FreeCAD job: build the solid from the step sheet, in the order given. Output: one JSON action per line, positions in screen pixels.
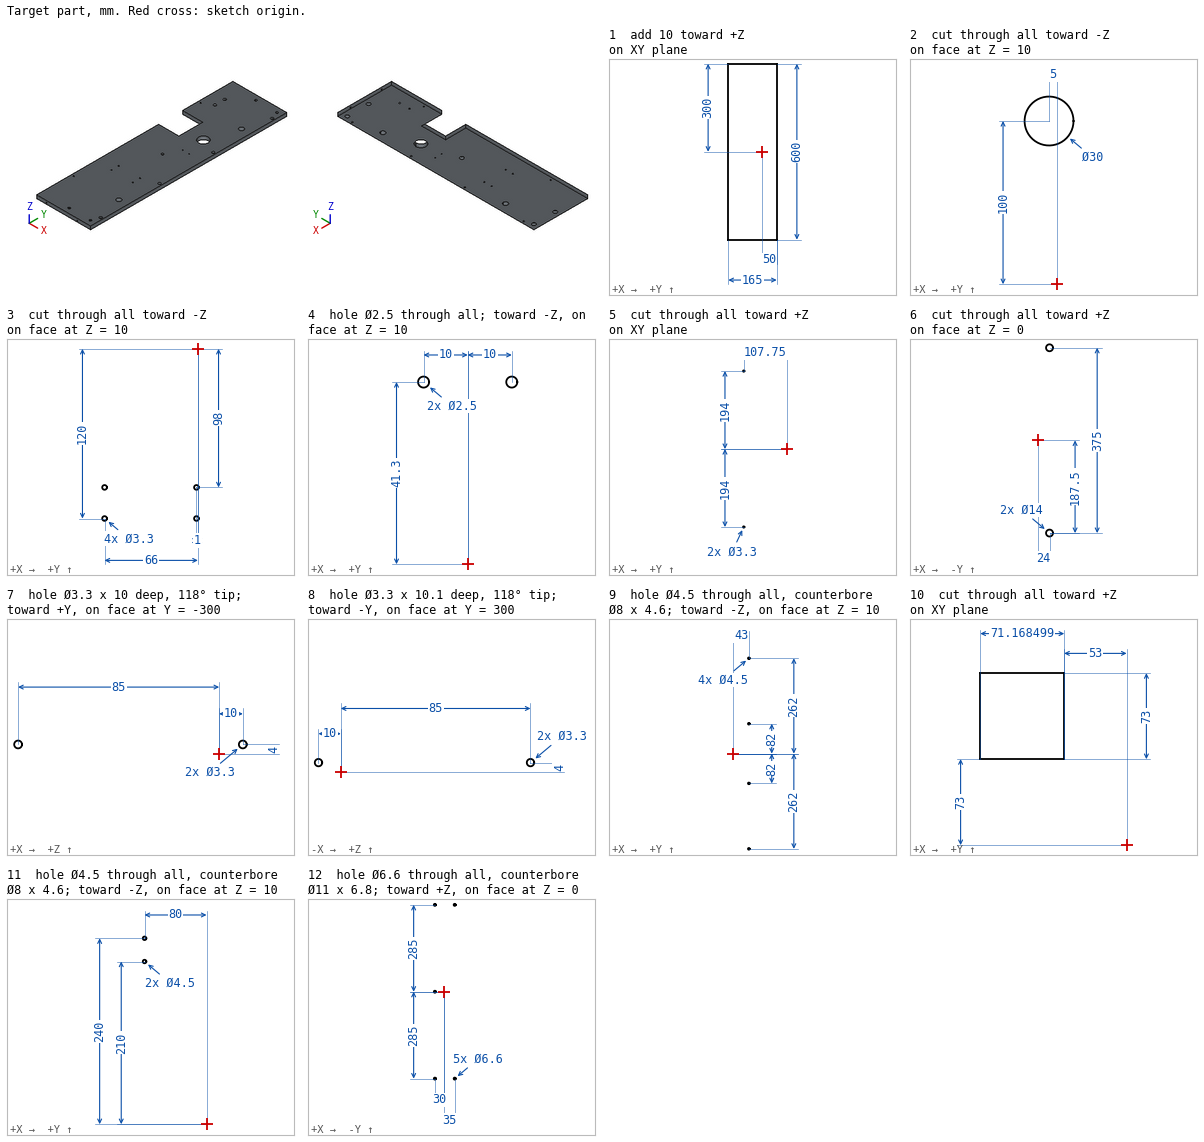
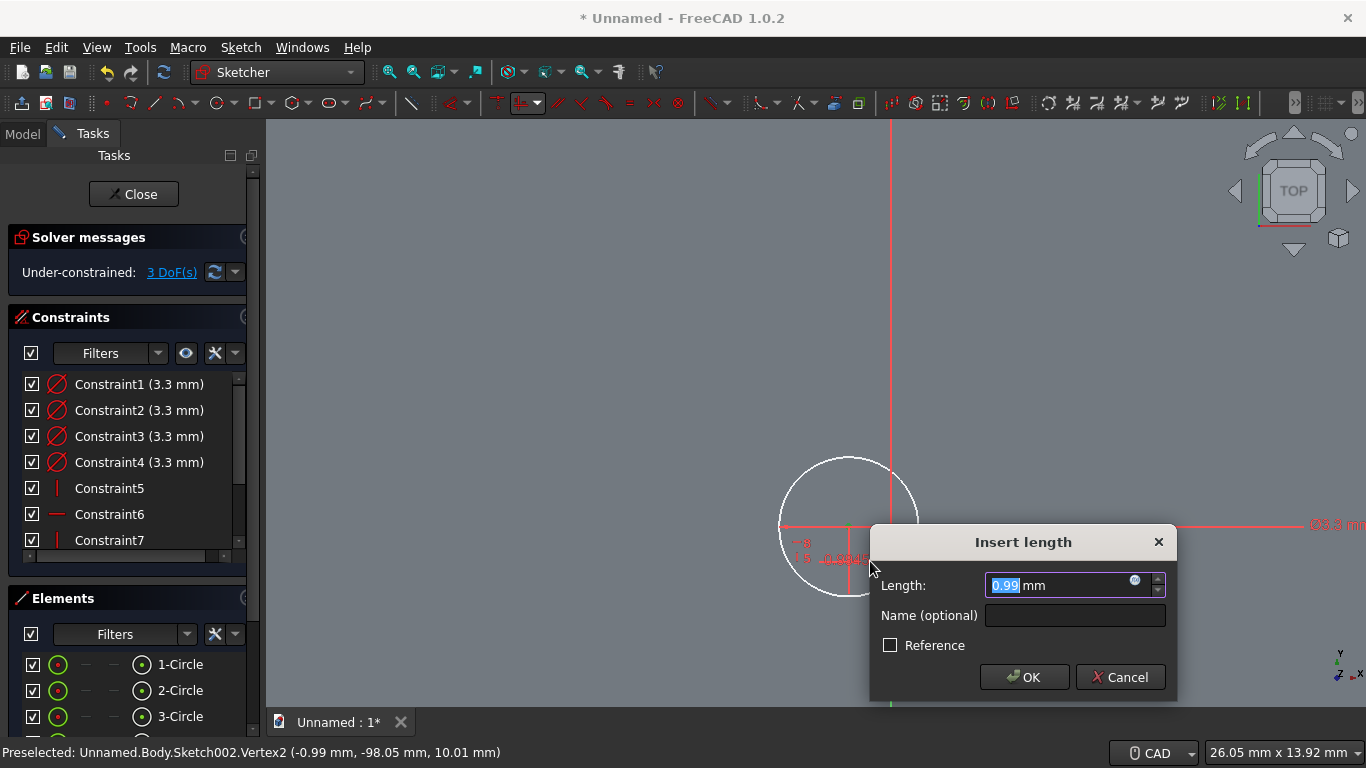
{"action": "type", "text": "1"}
{"action": "key", "text": "Return"}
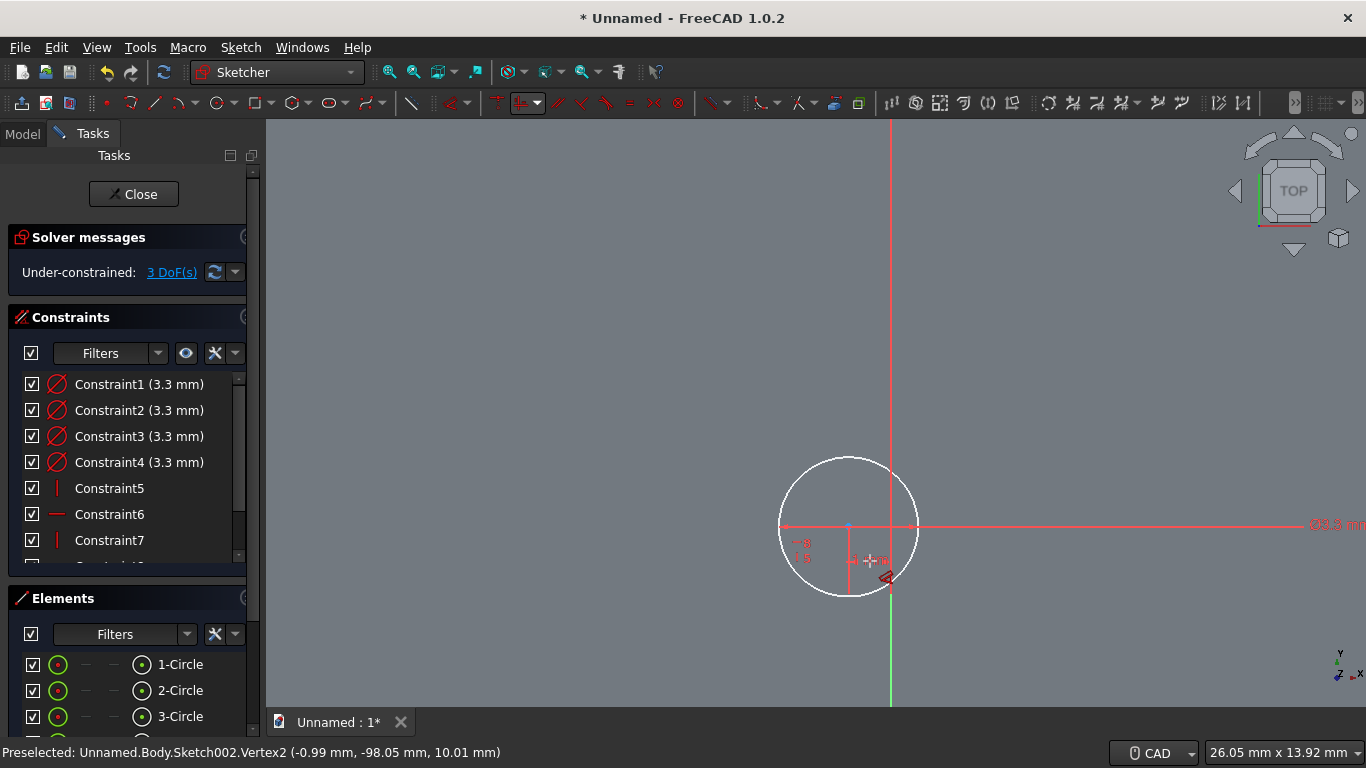
{"action": "scroll", "coordinate": [850, 530], "scroll_direction": "down", "scroll_amount": 13}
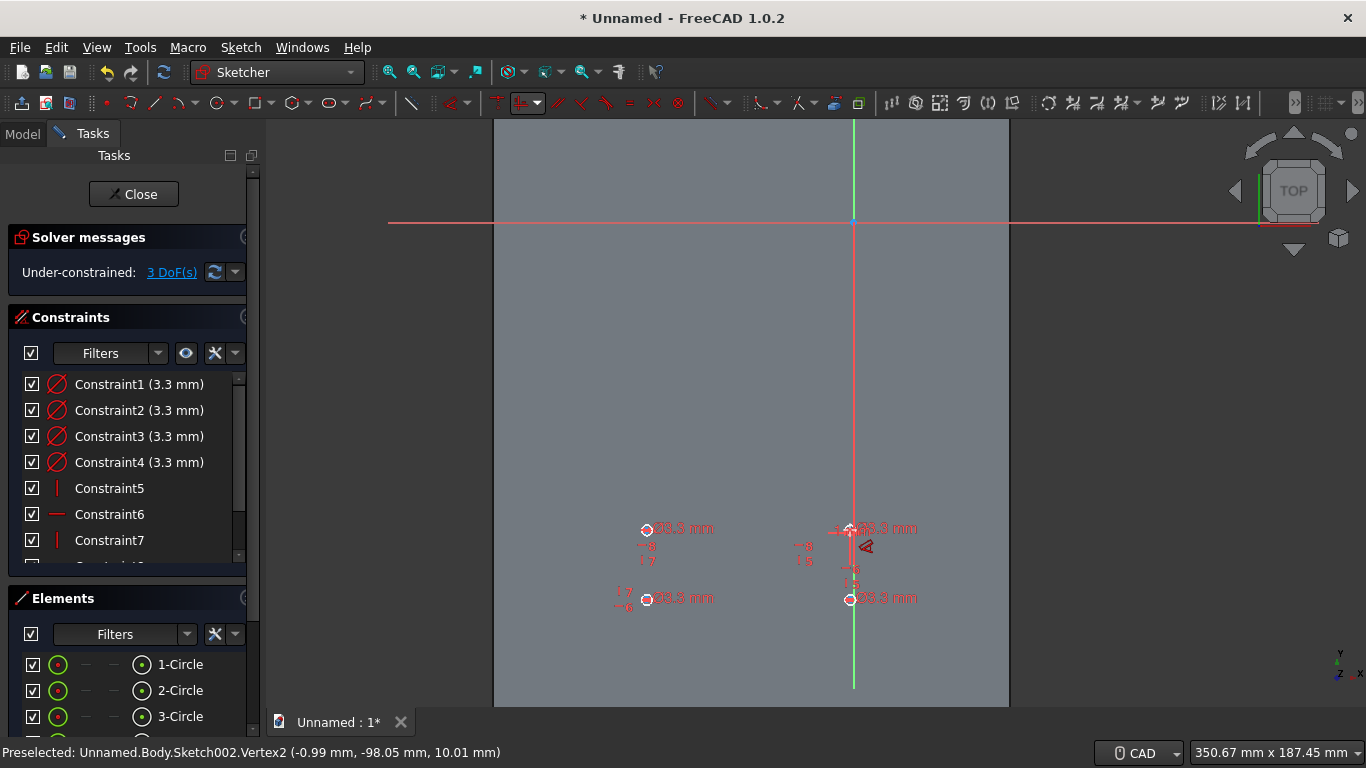
{"action": "left_click", "coordinate": [647, 600]}
{"action": "left_click", "coordinate": [750, 189]}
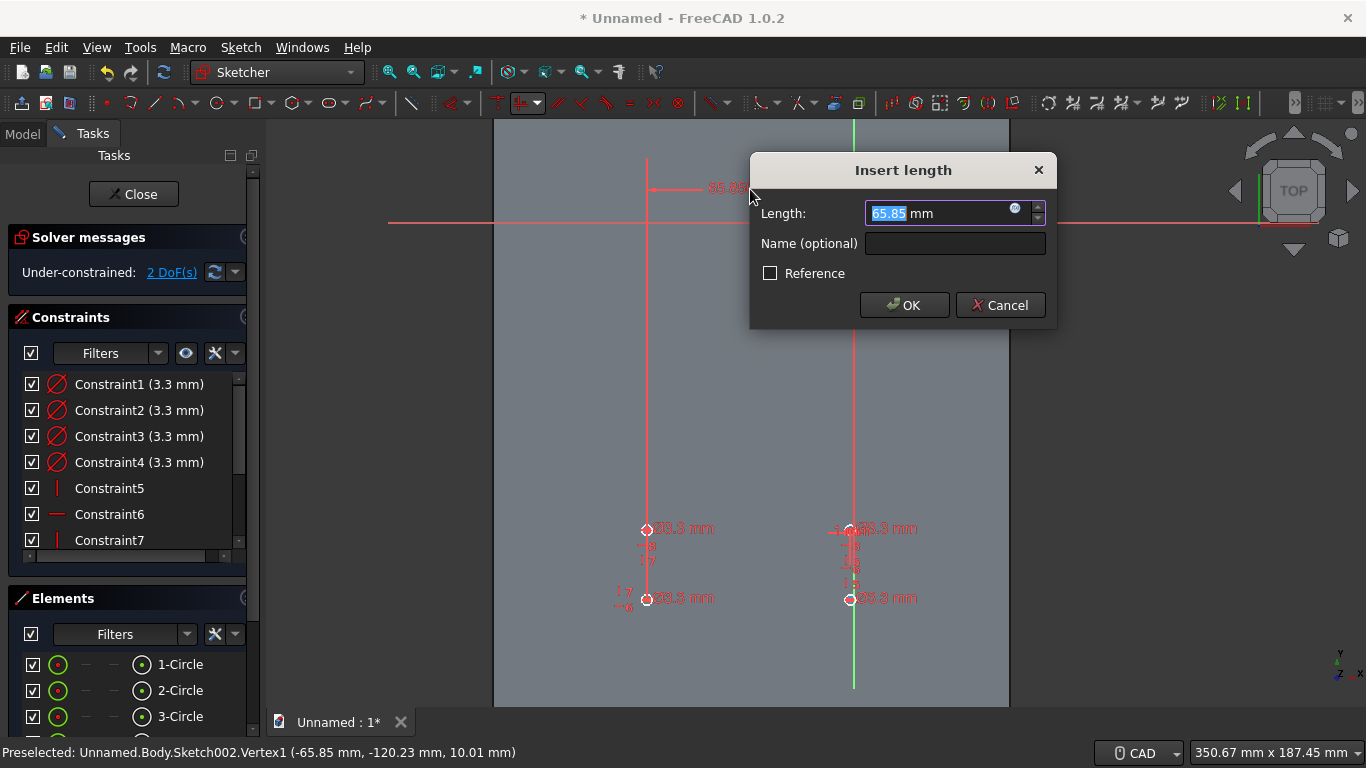
{"action": "type", "text": "66"}
{"action": "key", "text": "Return"}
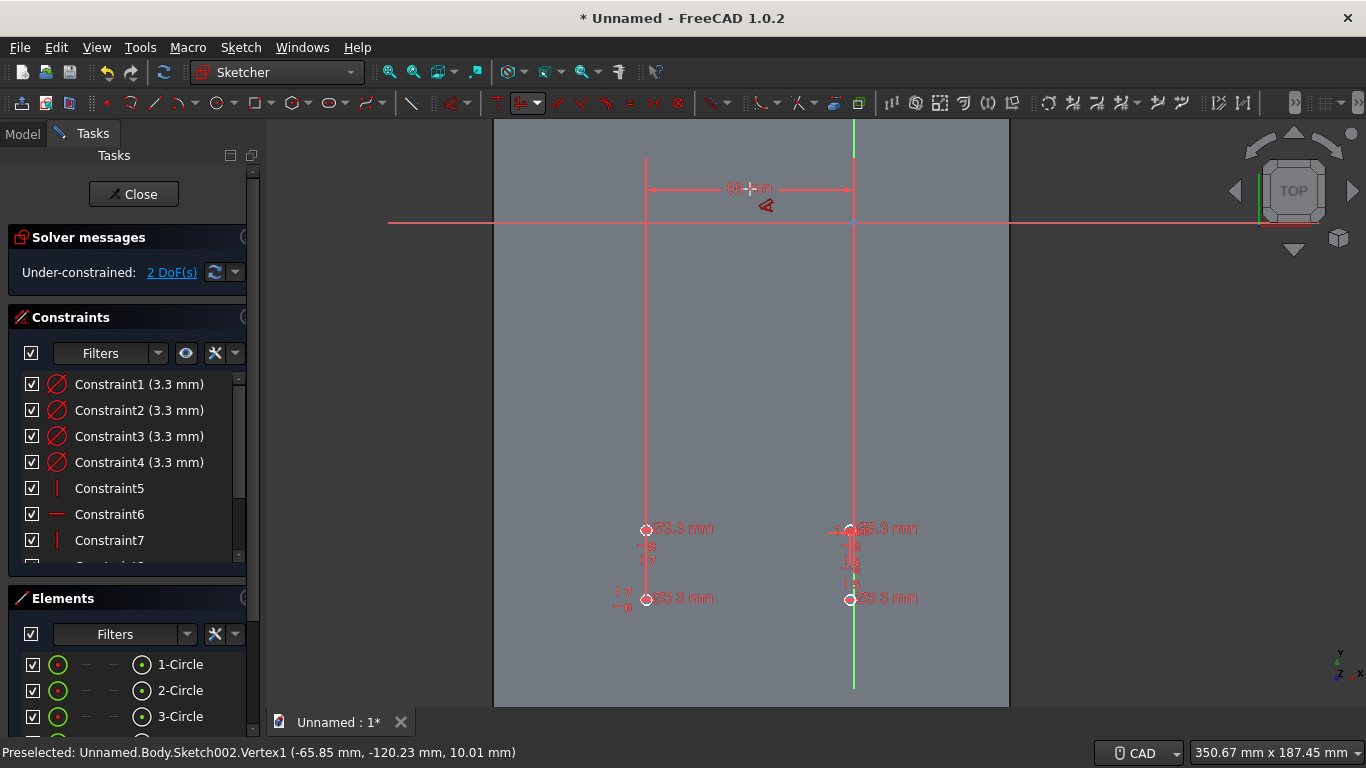
{"action": "left_click", "coordinate": [850, 530]}
{"action": "left_click", "coordinate": [888, 377]}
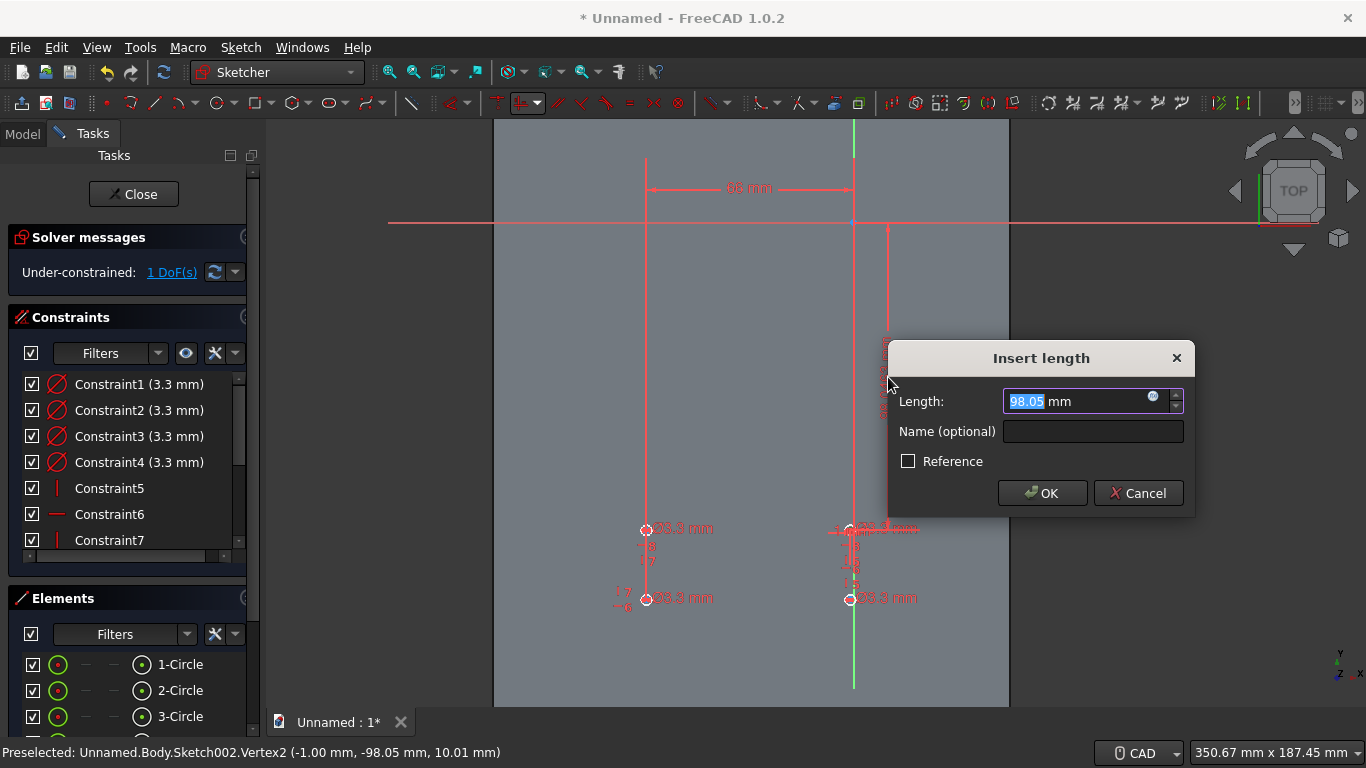
{"action": "type", "text": "98"}
{"action": "key", "text": "Return"}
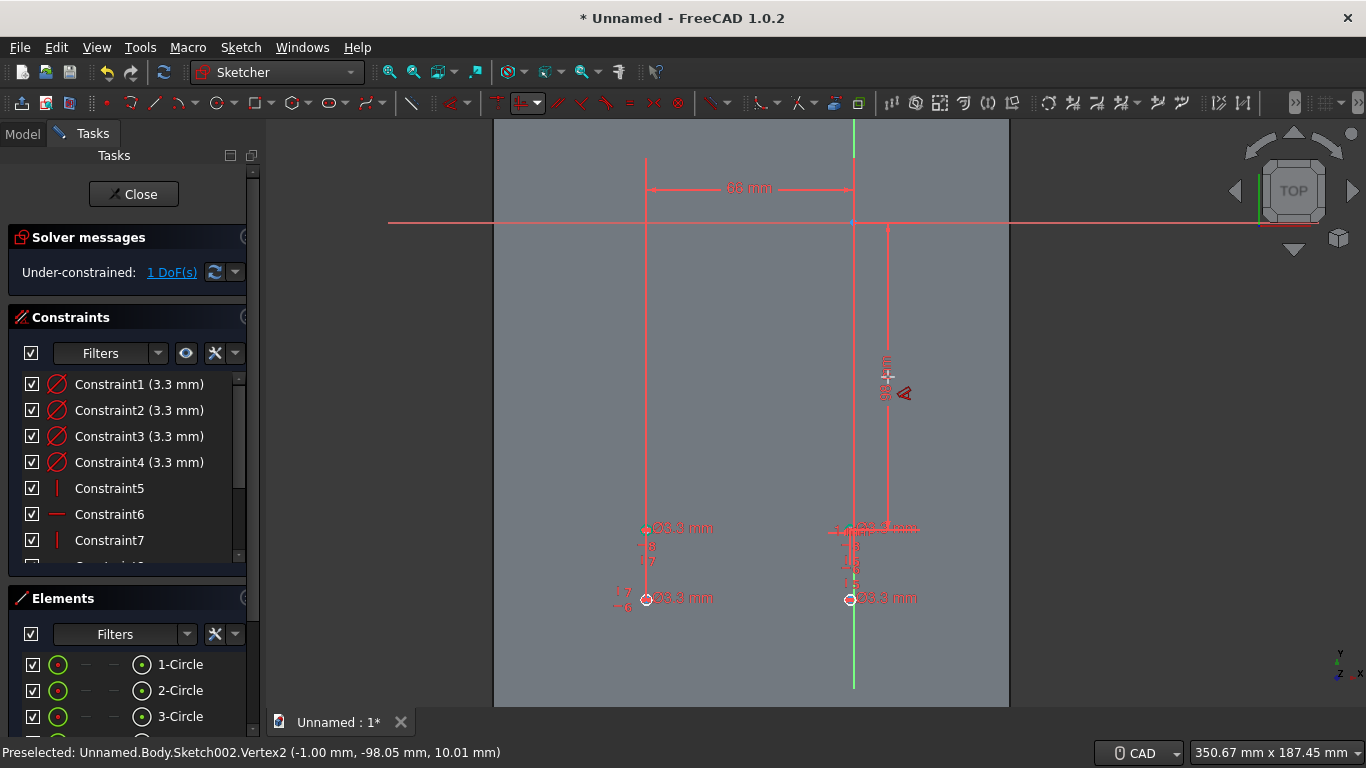
{"action": "left_click", "coordinate": [646, 600]}
{"action": "left_click", "coordinate": [888, 411]}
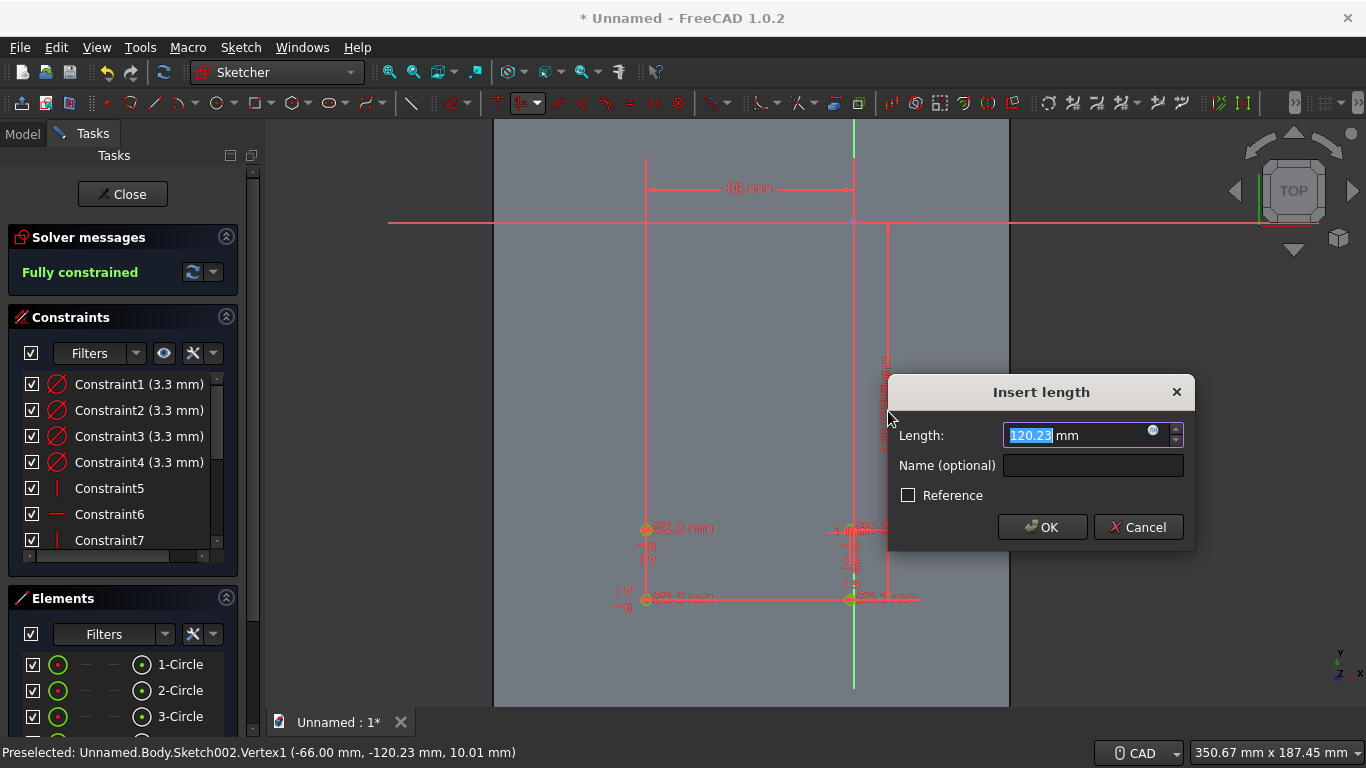
{"action": "type", "text": "120"}
{"action": "key", "text": "Return"}
{"action": "key", "text": "Escape"}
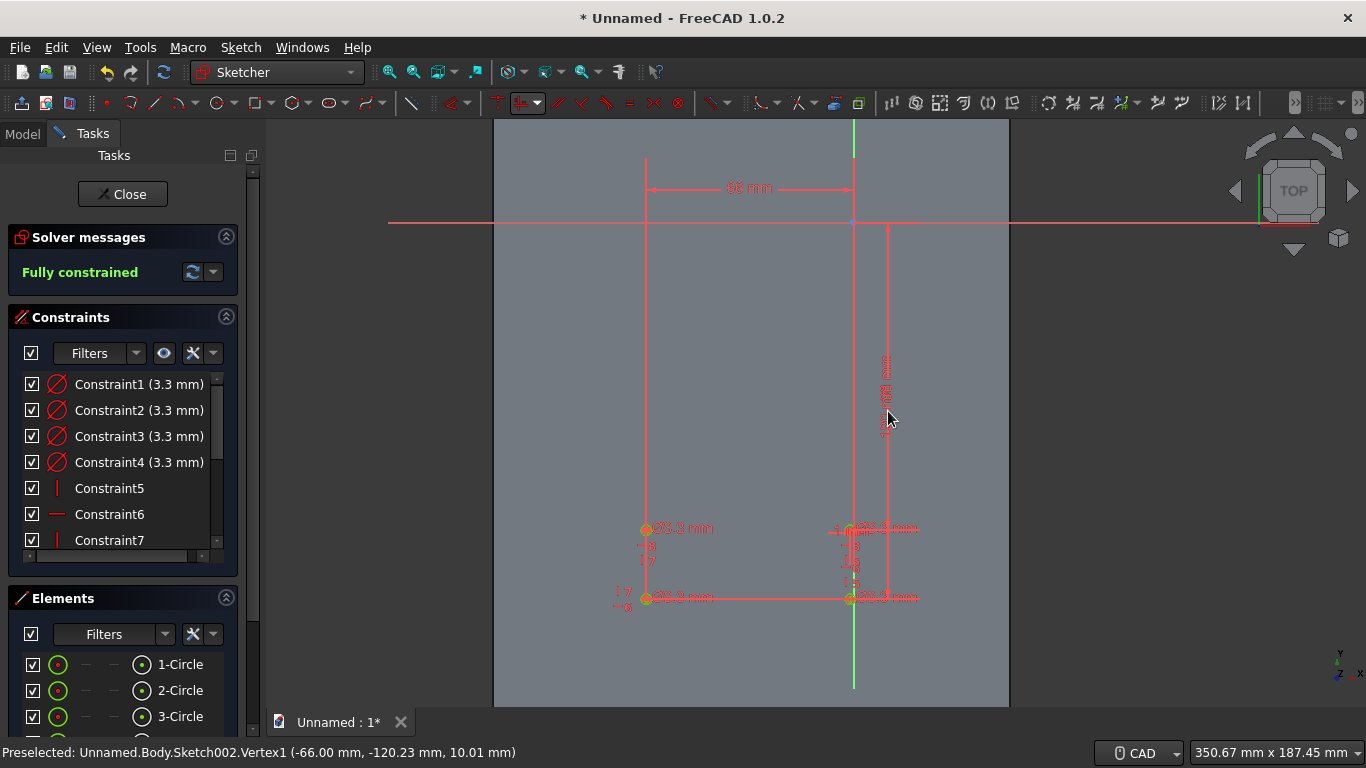
{"action": "left_click", "coordinate": [123, 194]}